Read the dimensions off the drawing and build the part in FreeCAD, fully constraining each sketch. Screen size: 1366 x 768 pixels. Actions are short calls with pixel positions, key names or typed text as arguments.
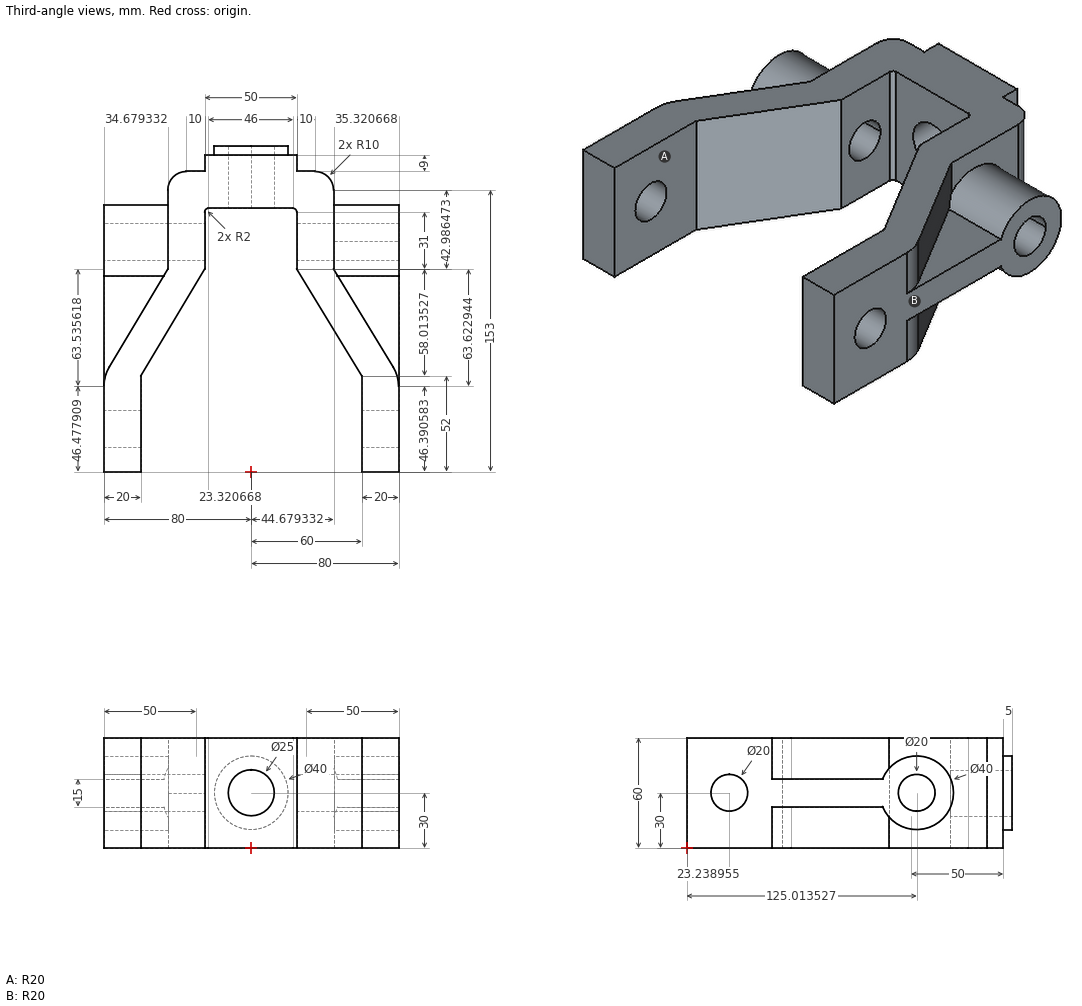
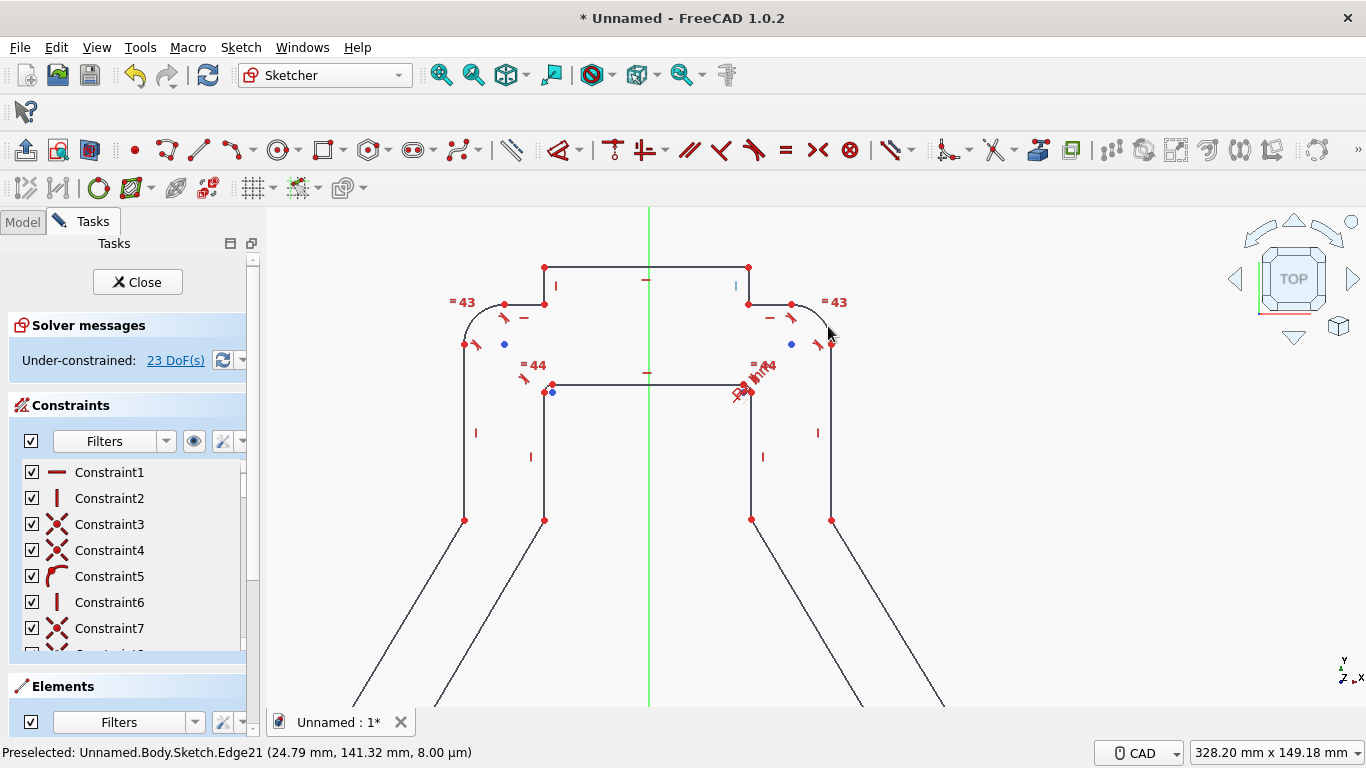
click(827, 327)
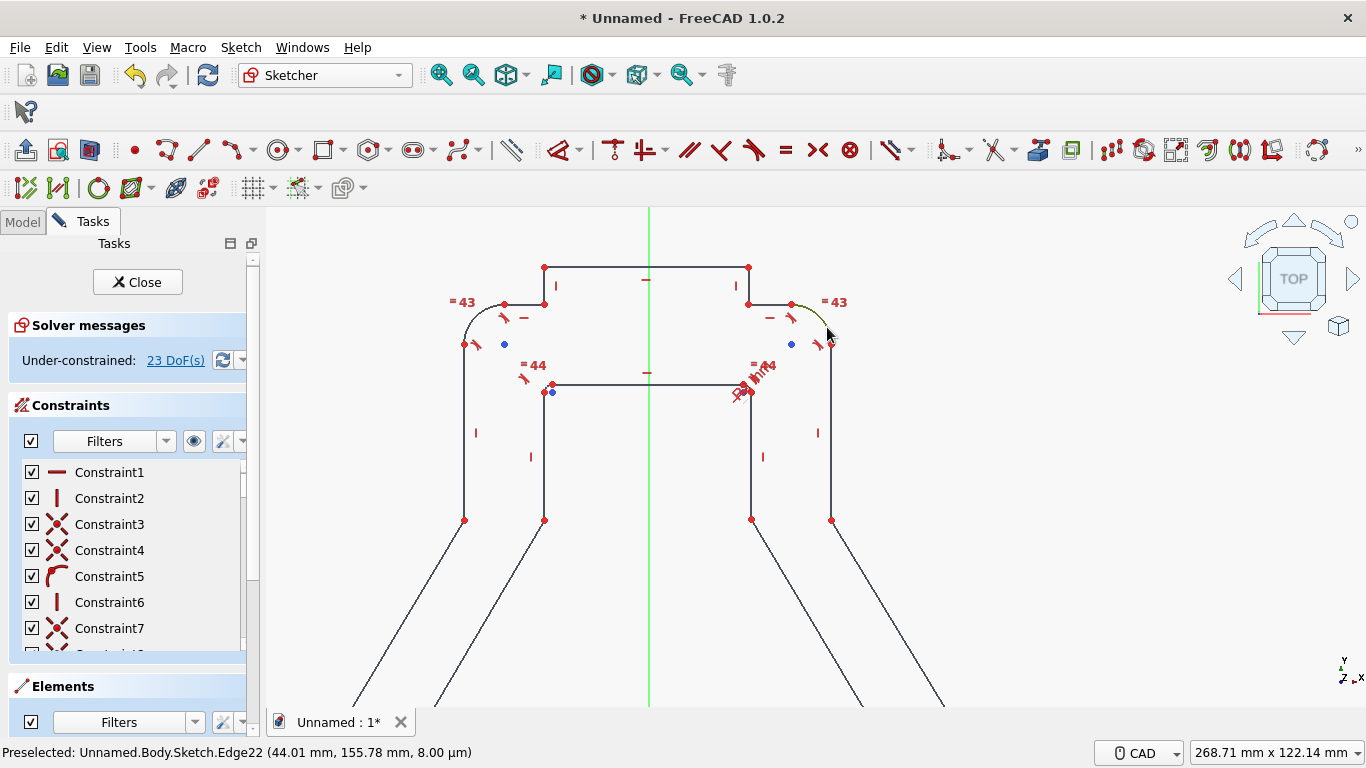
key(k)
key(r)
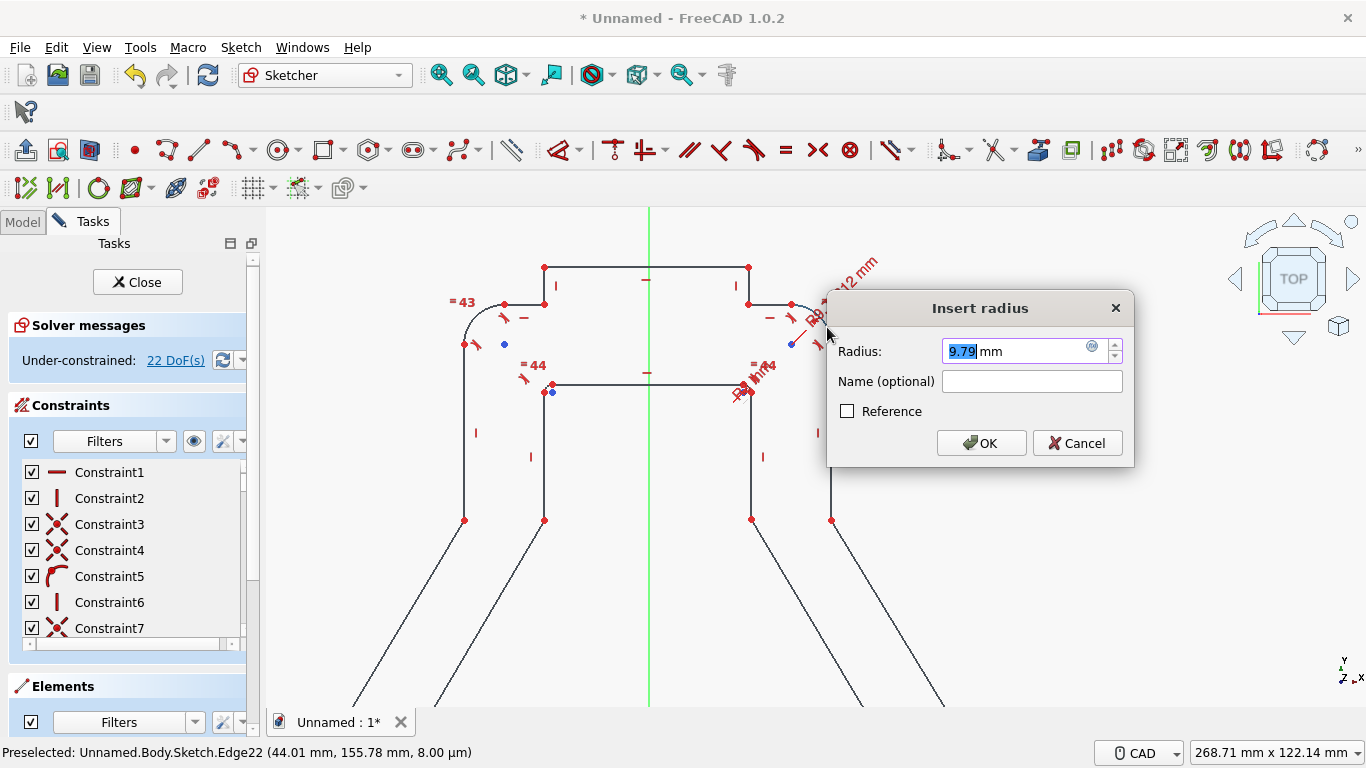
text(10)
key(Return)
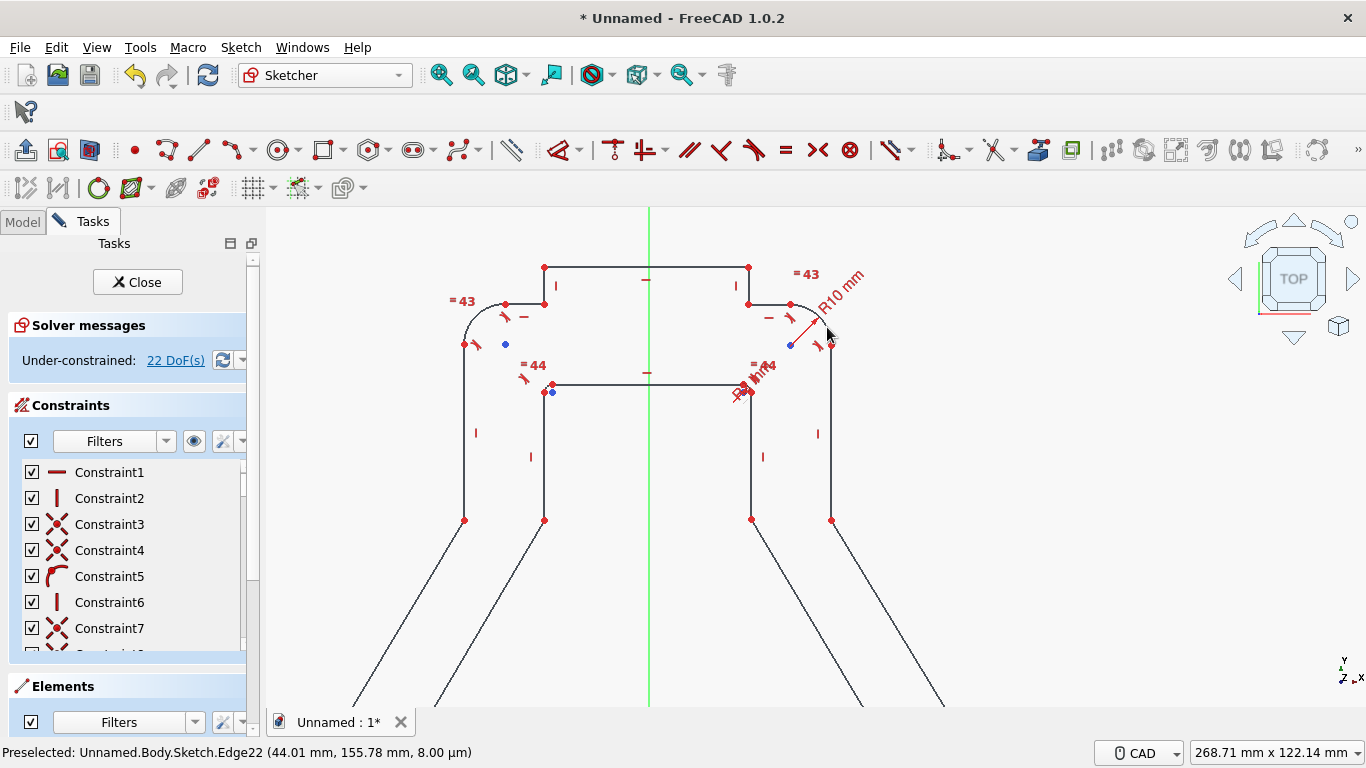
click(749, 293)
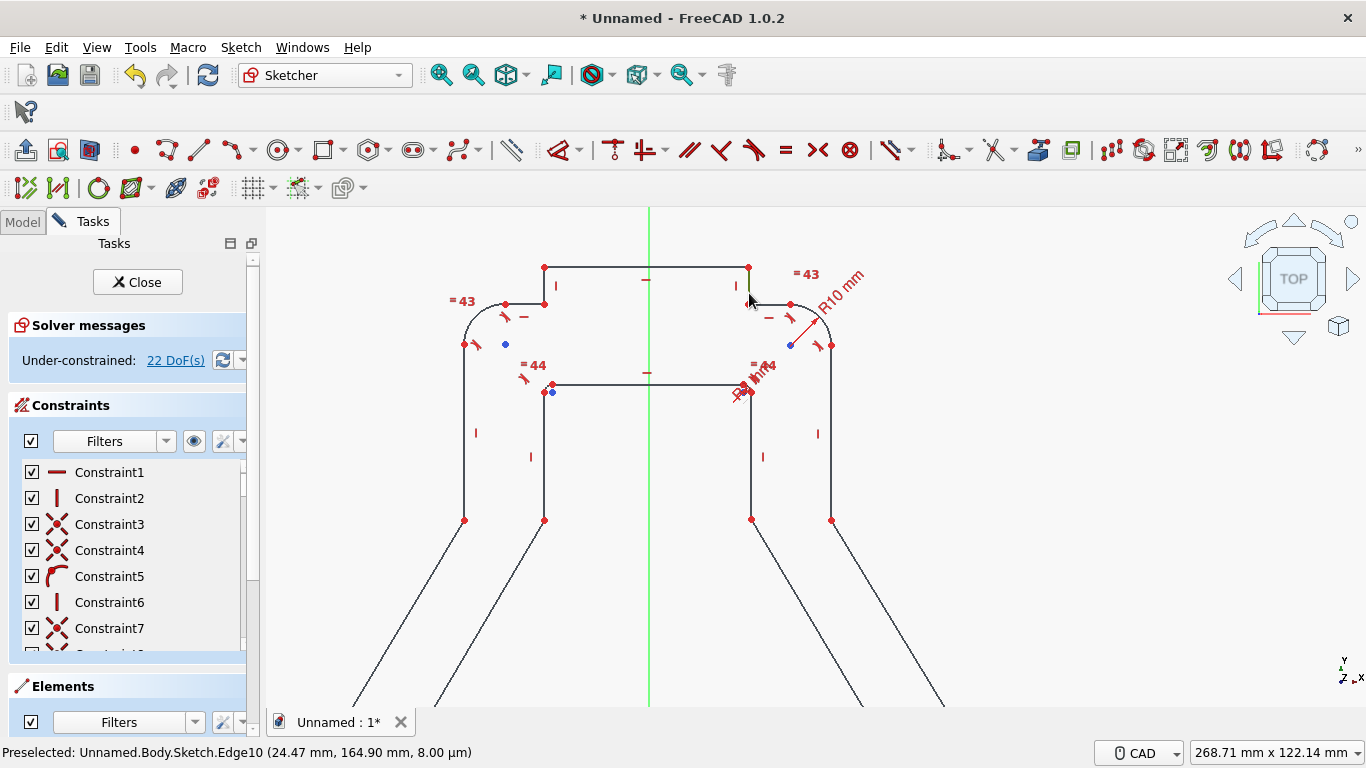
key(i)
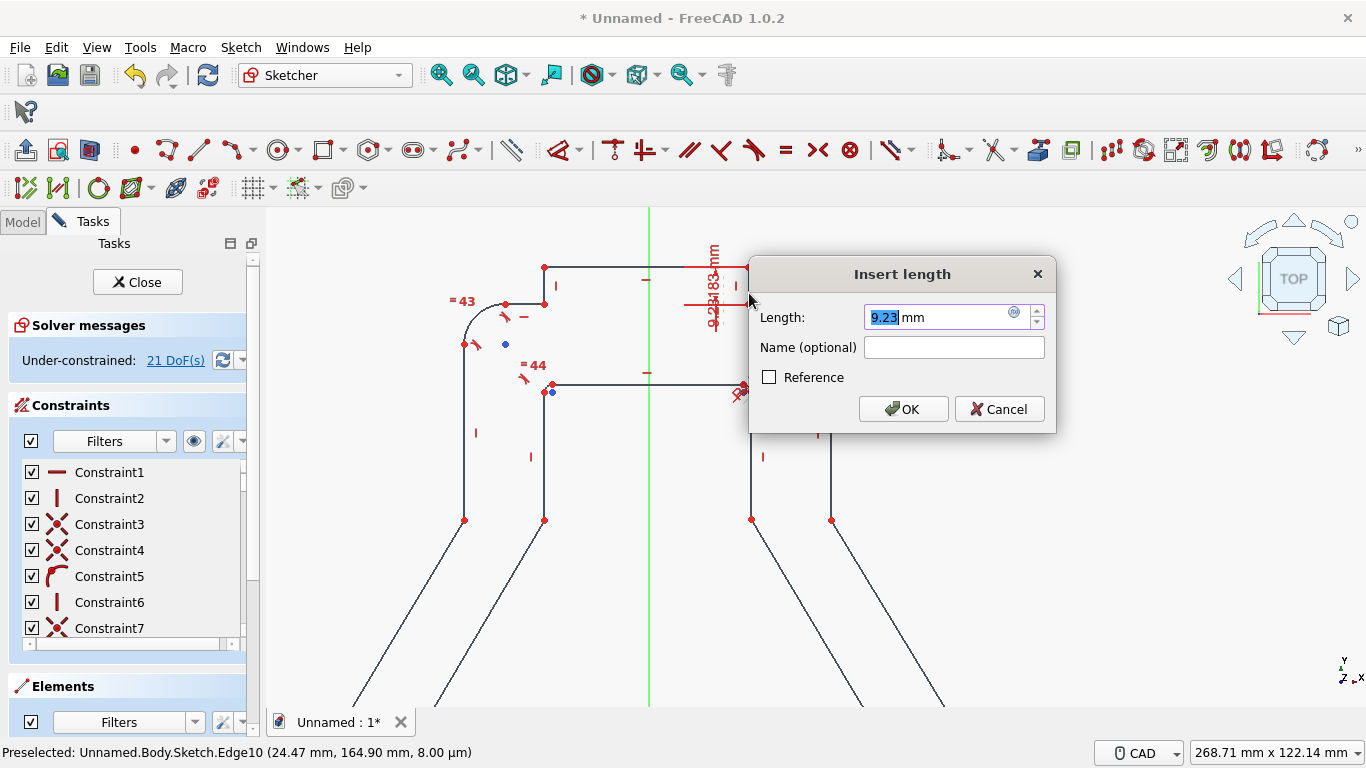
text(9)
key(Return)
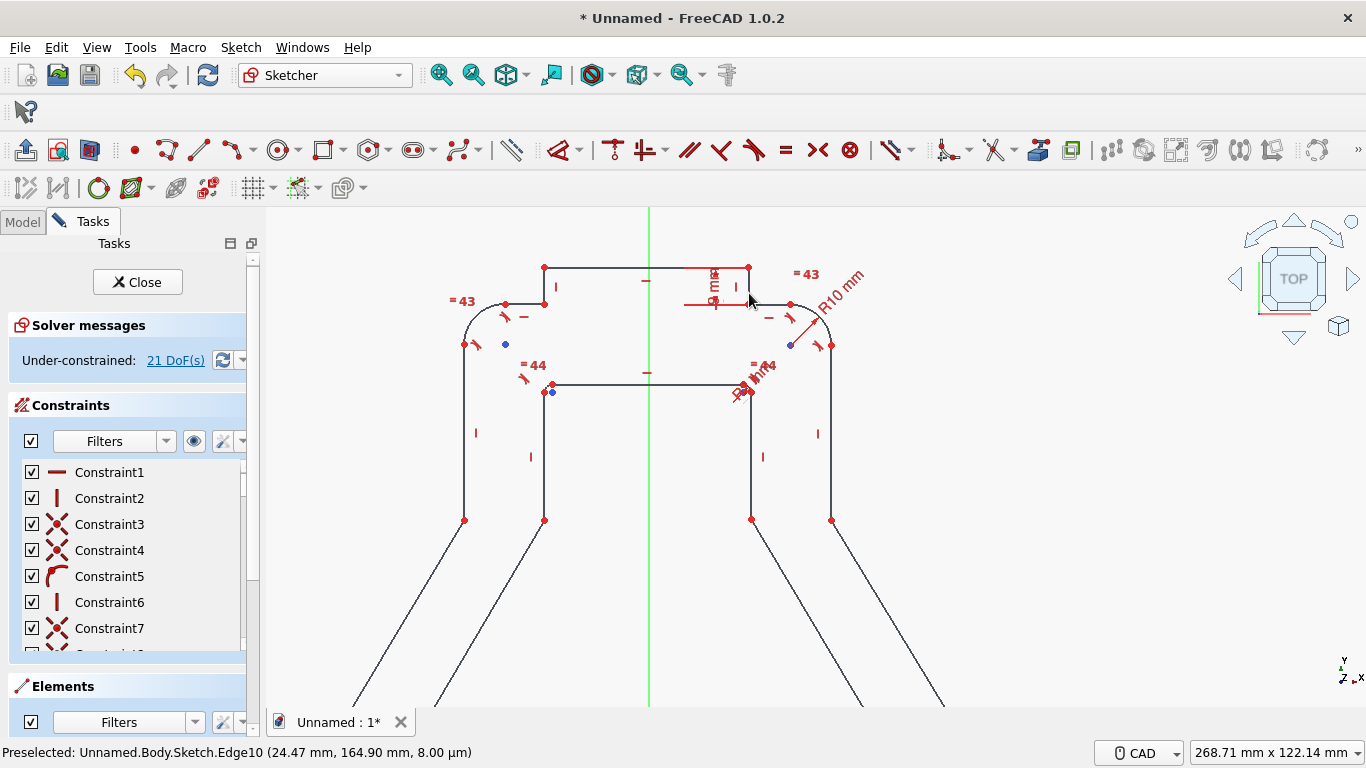
scroll(544, 279, up, 2)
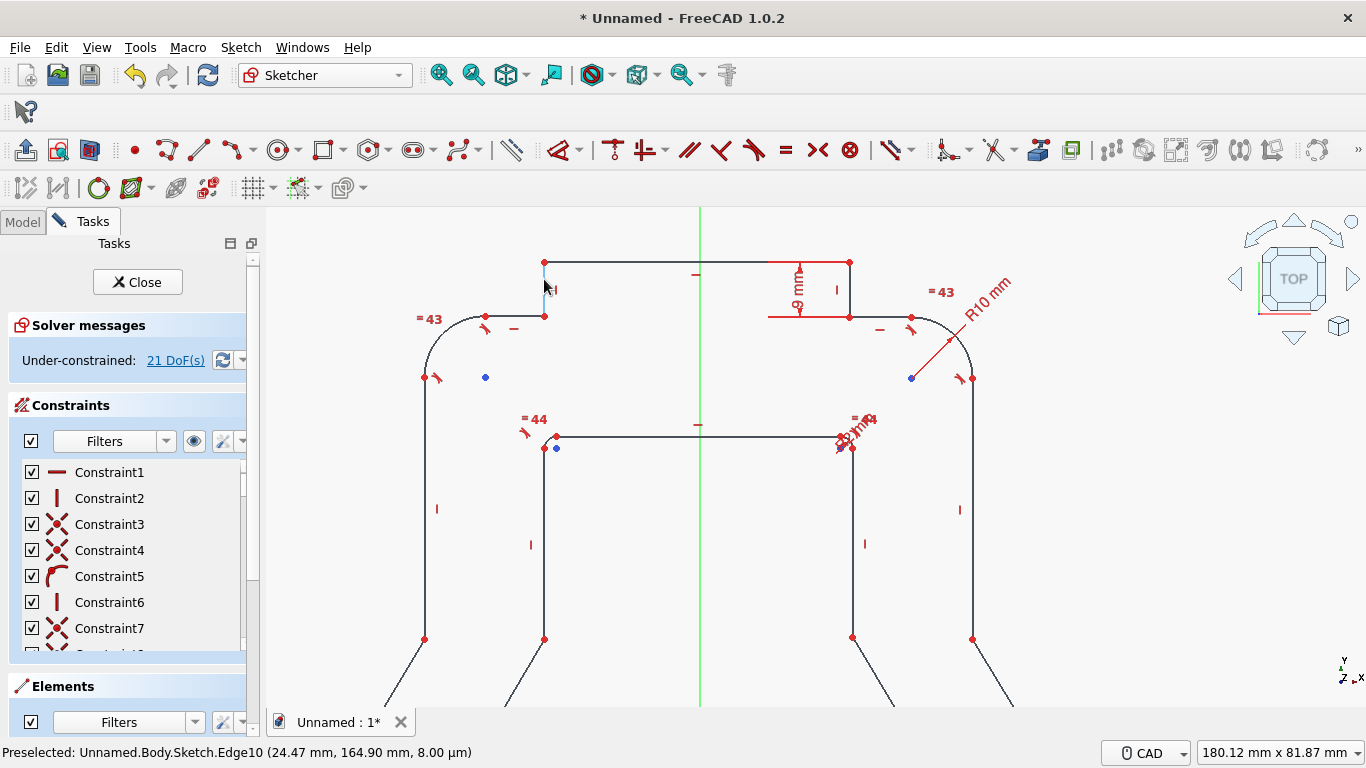
click(544, 279)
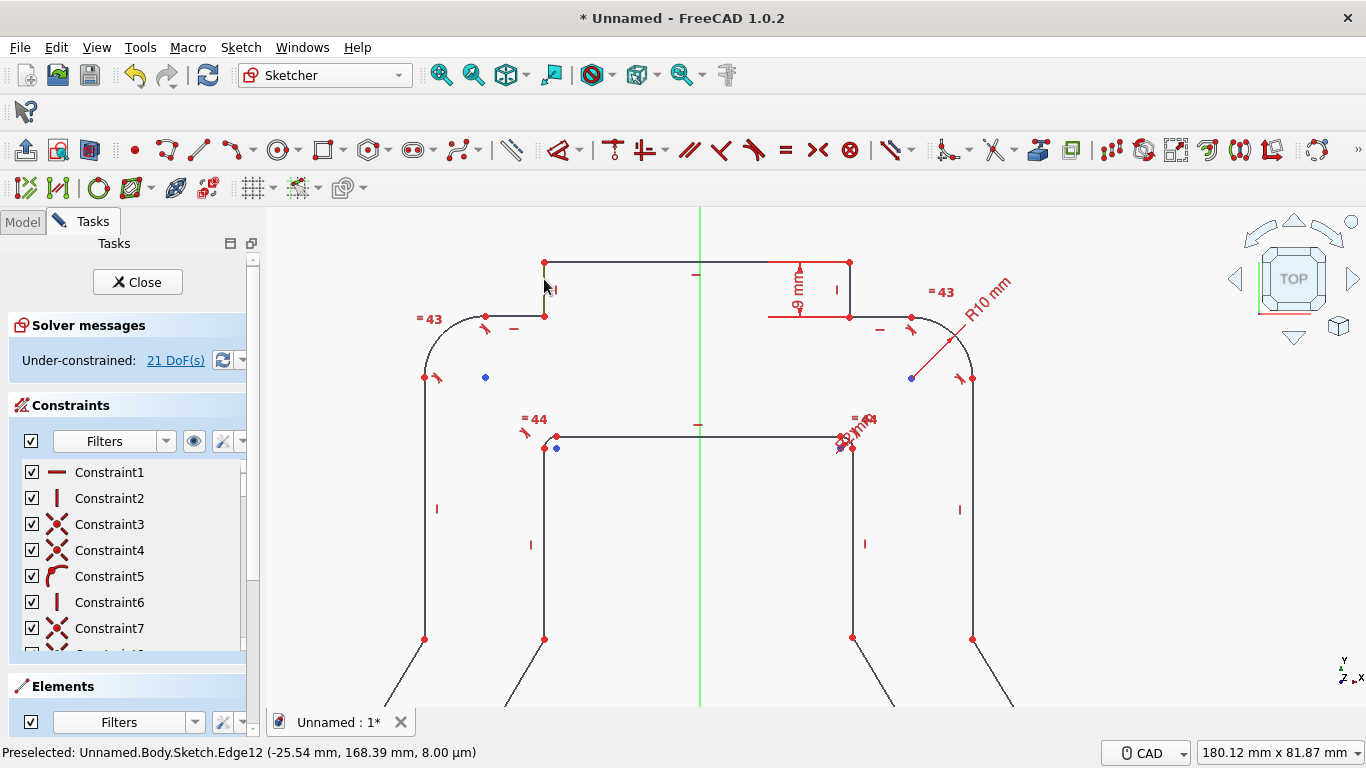
key(i)